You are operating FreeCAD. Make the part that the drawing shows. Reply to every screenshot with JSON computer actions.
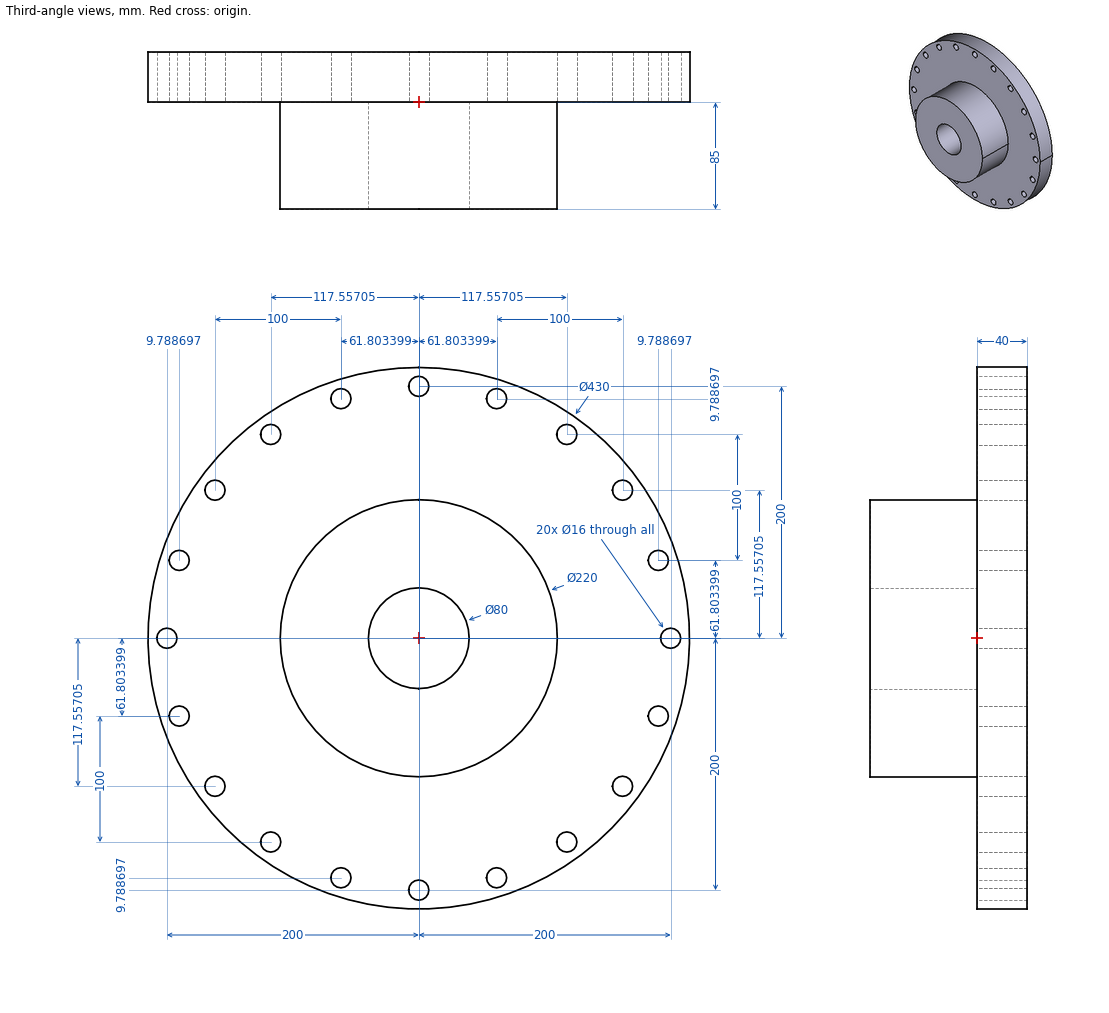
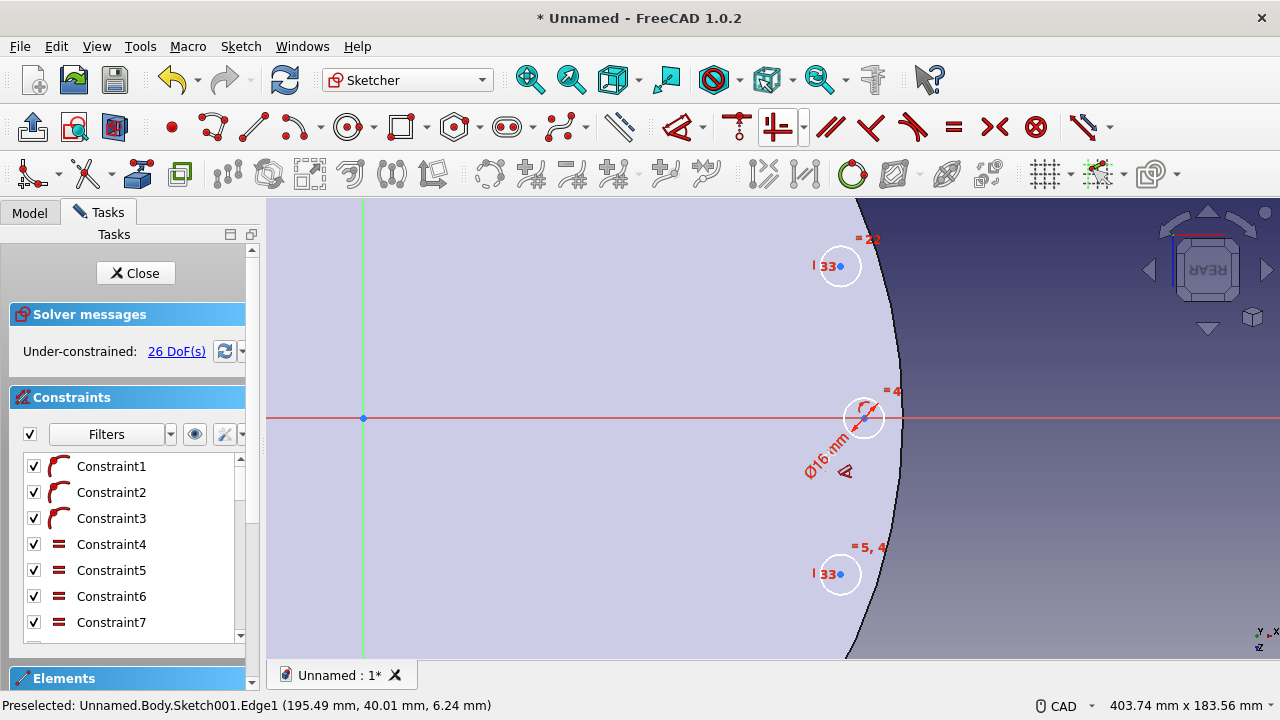
{"action": "left_click", "coordinate": [864, 418]}
{"action": "left_click", "coordinate": [614, 452]}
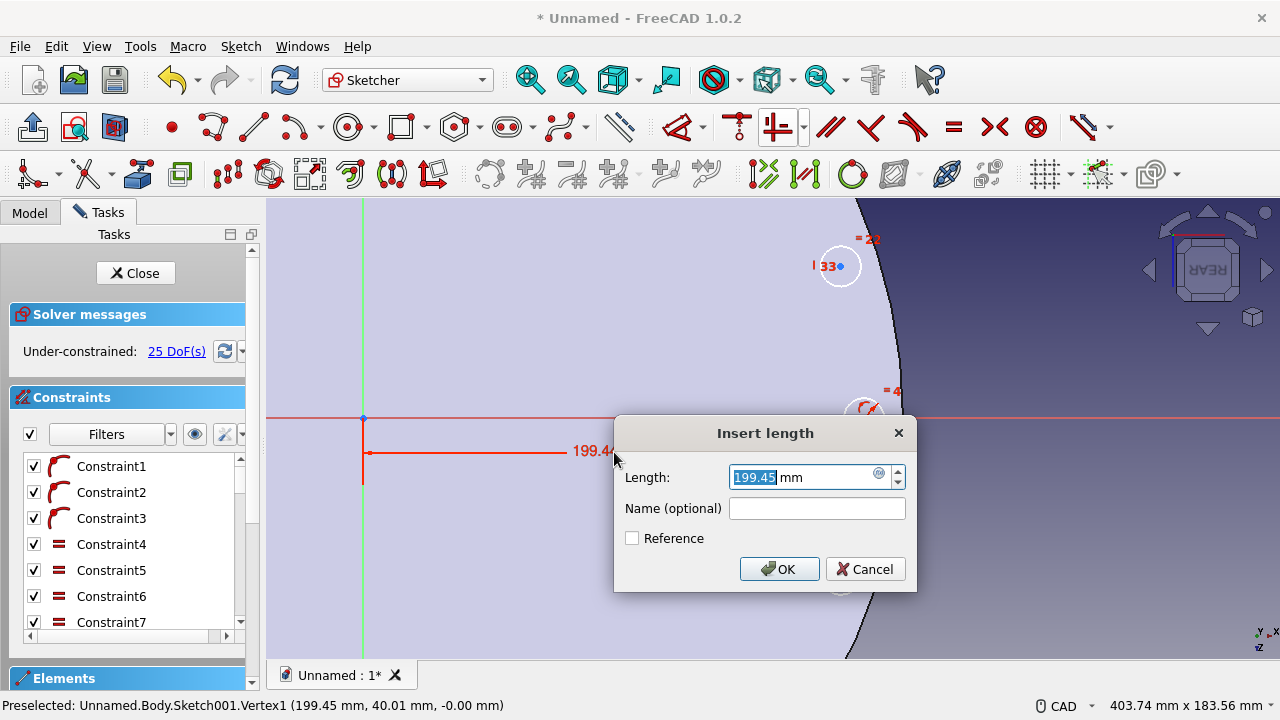
{"action": "type", "text": "200"}
{"action": "key", "text": "Return"}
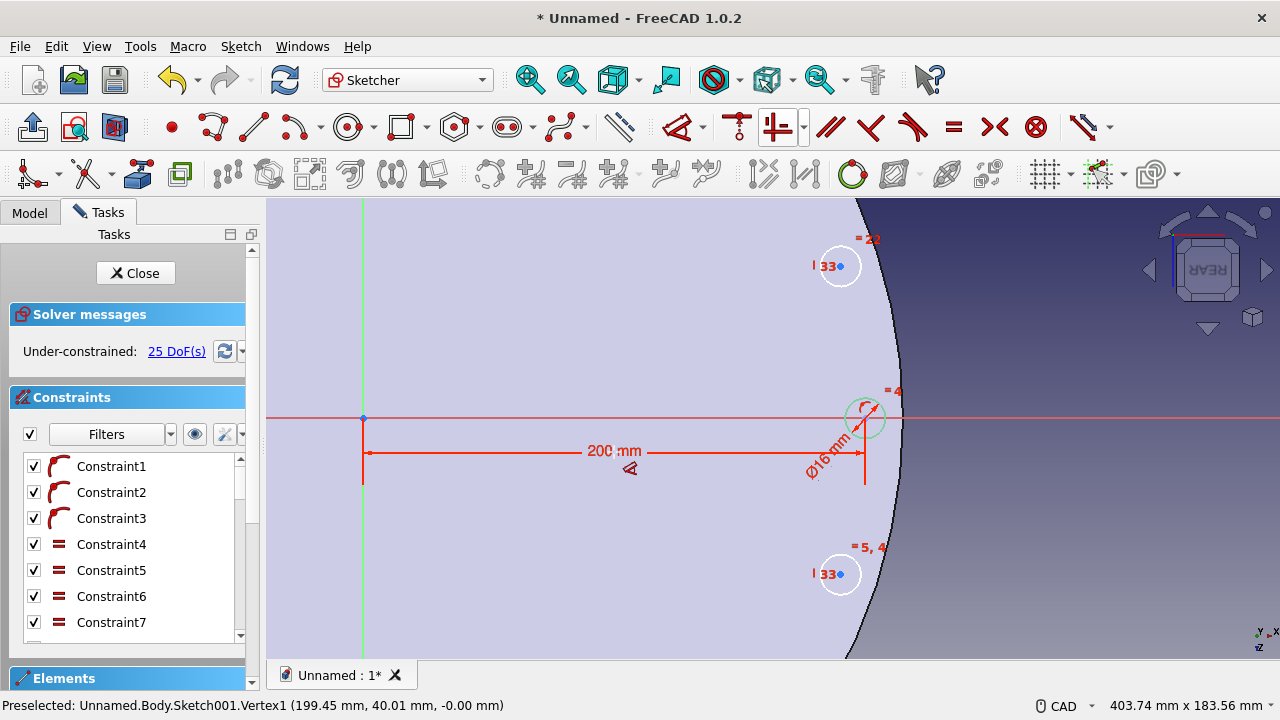
{"action": "scroll", "coordinate": [852, 433], "scroll_direction": "down", "scroll_amount": 6}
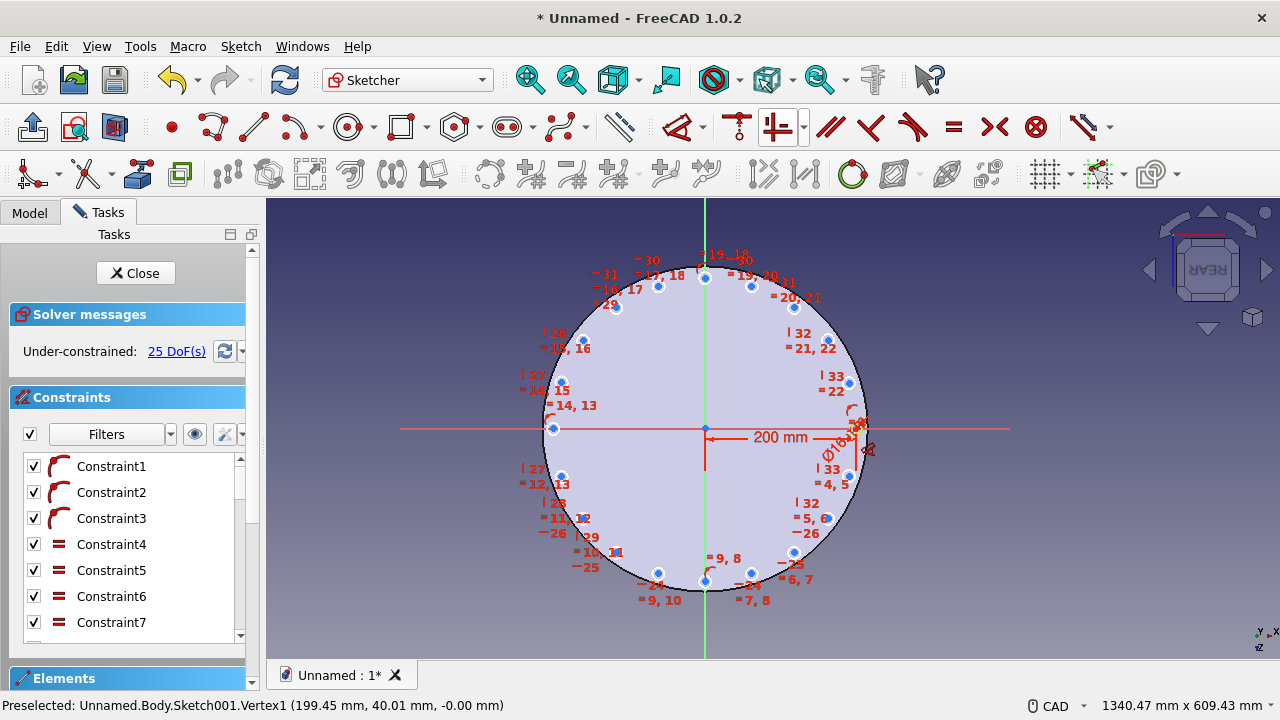
{"action": "left_click", "coordinate": [705, 582]}
{"action": "left_click", "coordinate": [739, 505]}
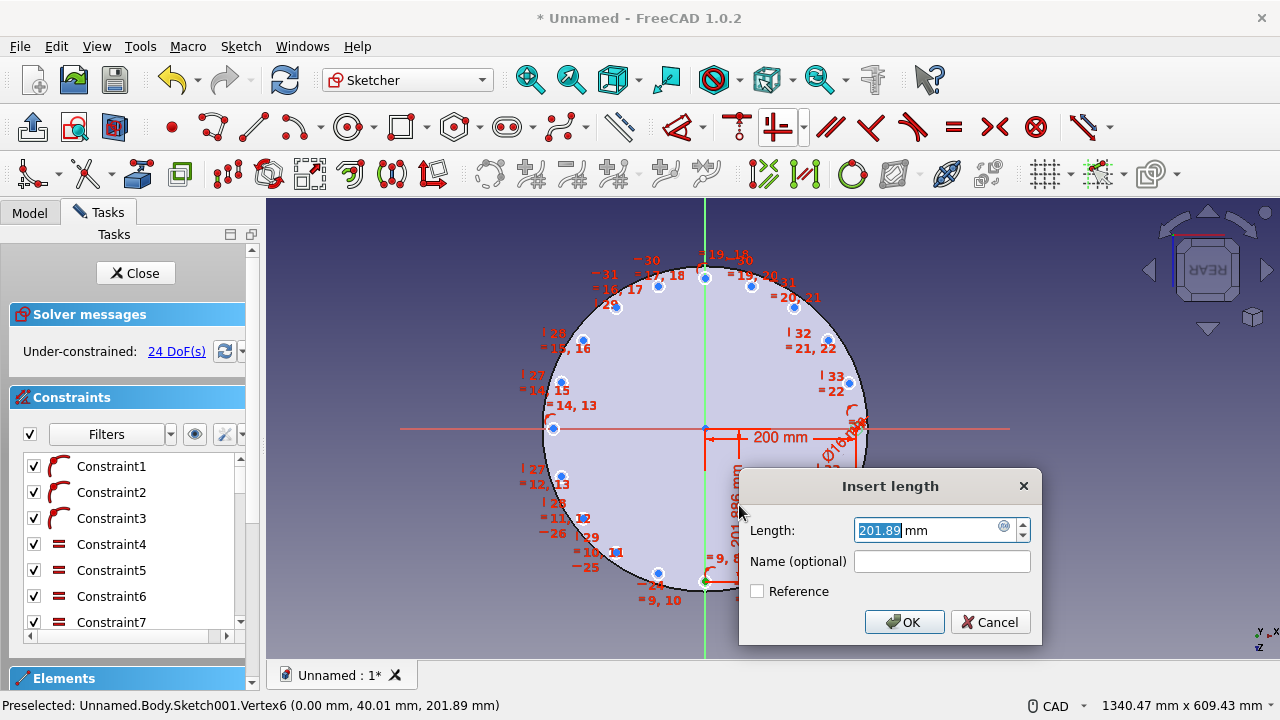
{"action": "type", "text": "200"}
{"action": "key", "text": "Return"}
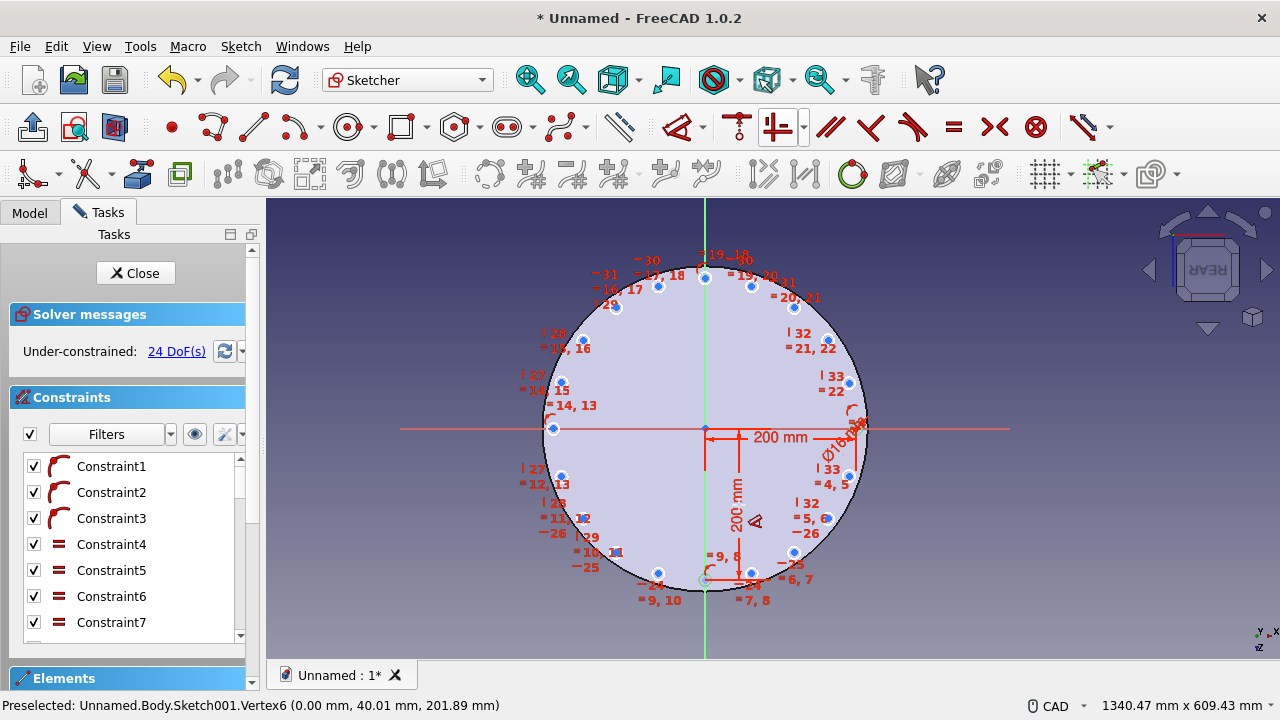
{"action": "left_click", "coordinate": [553, 429]}
{"action": "left_click", "coordinate": [629, 463]}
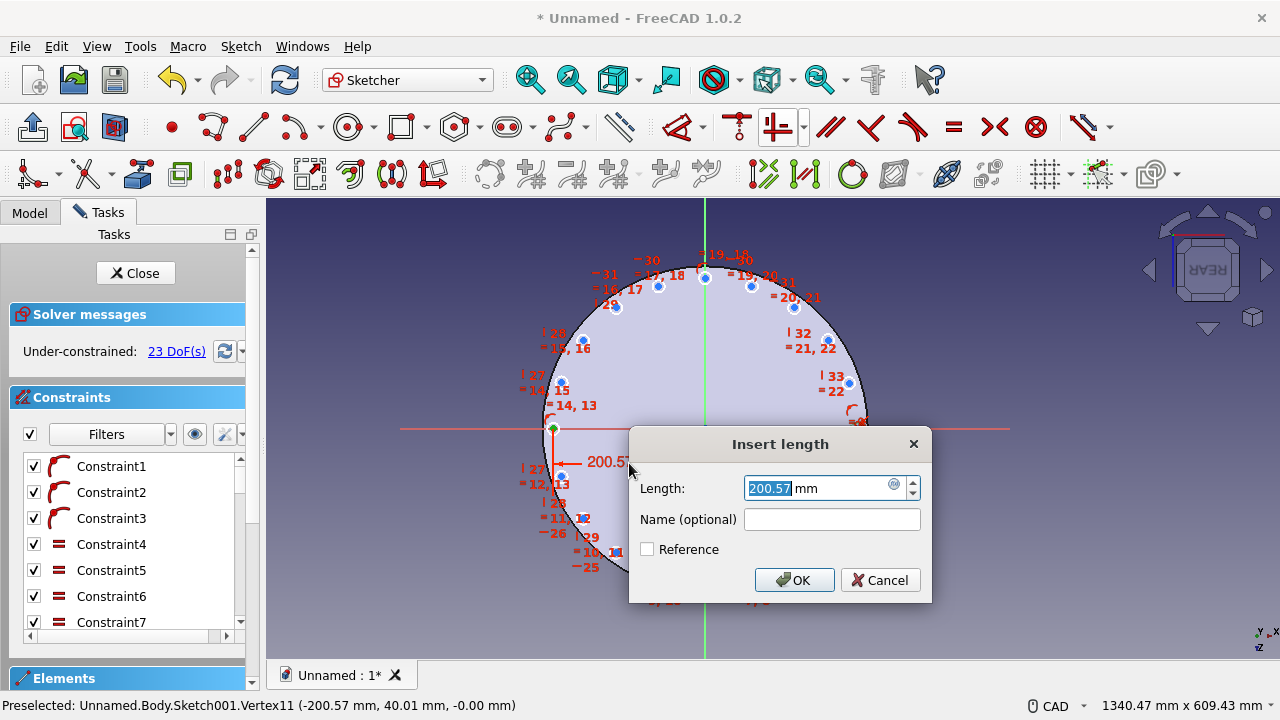
{"action": "type", "text": "200"}
{"action": "key", "text": "Return"}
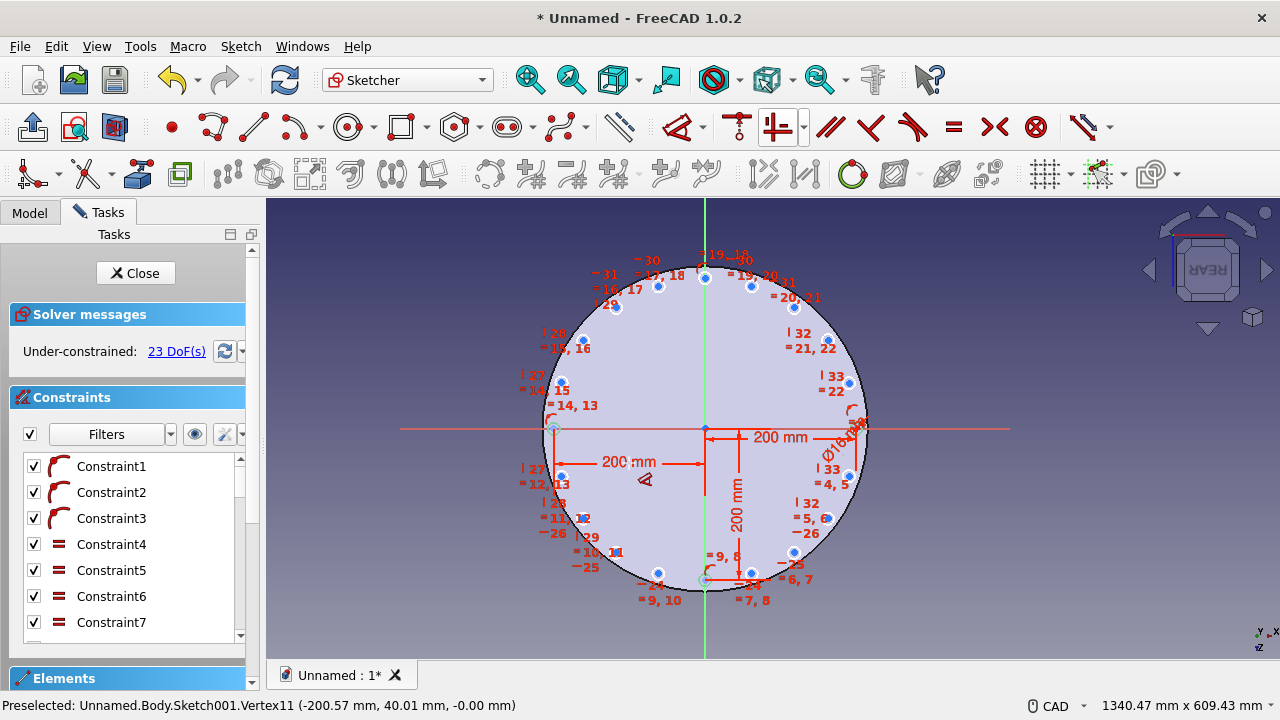
{"action": "left_click", "coordinate": [705, 278]}
{"action": "left_click", "coordinate": [739, 354]}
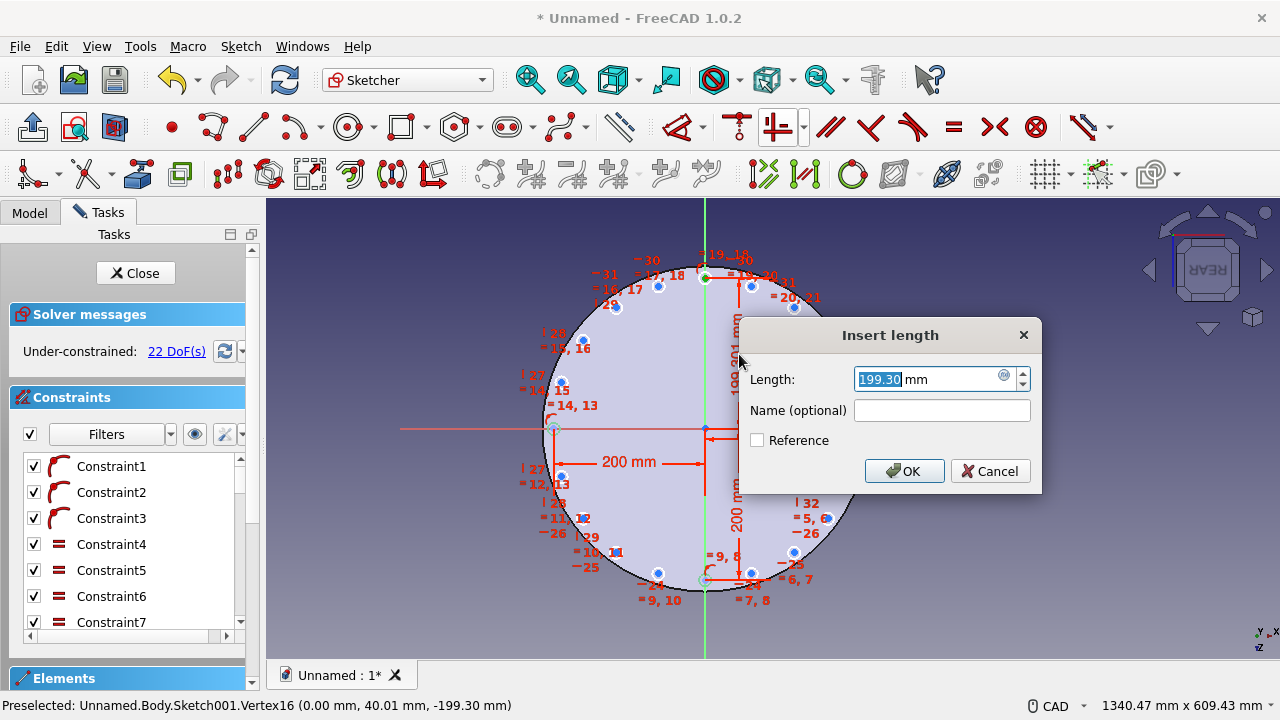
{"action": "type", "text": "200"}
{"action": "key", "text": "Return"}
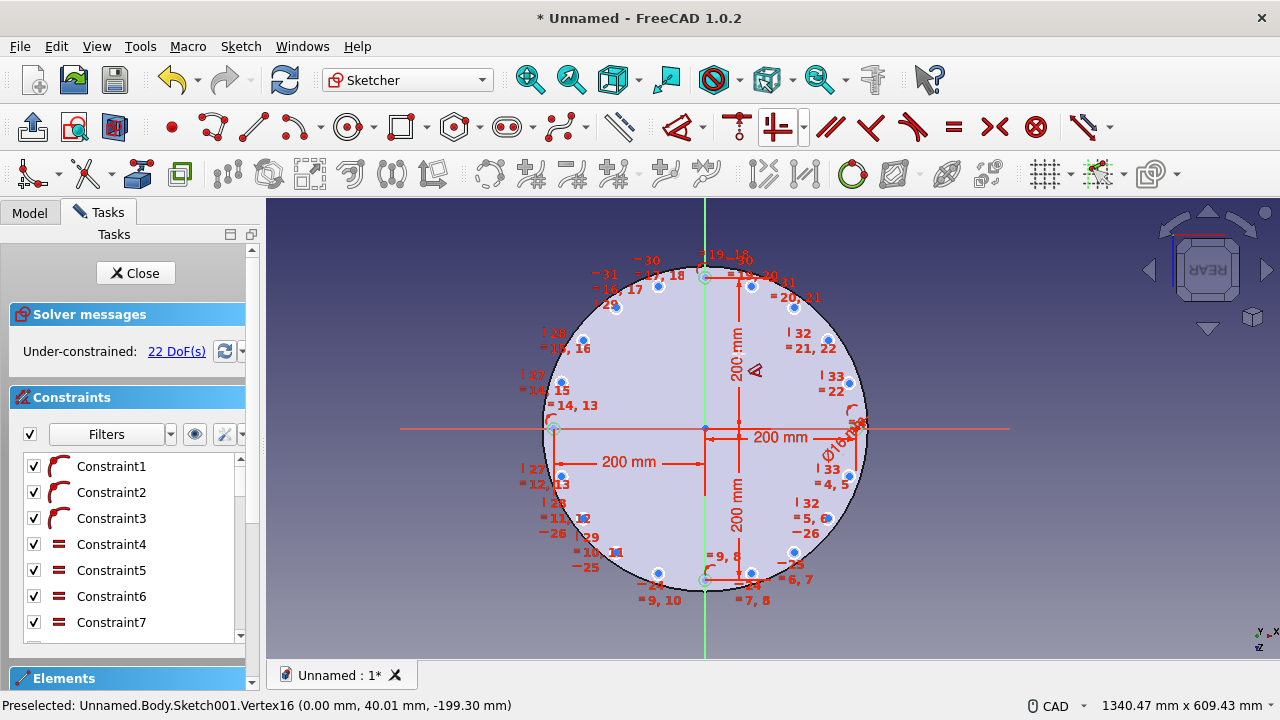
{"action": "left_click", "coordinate": [849, 476]}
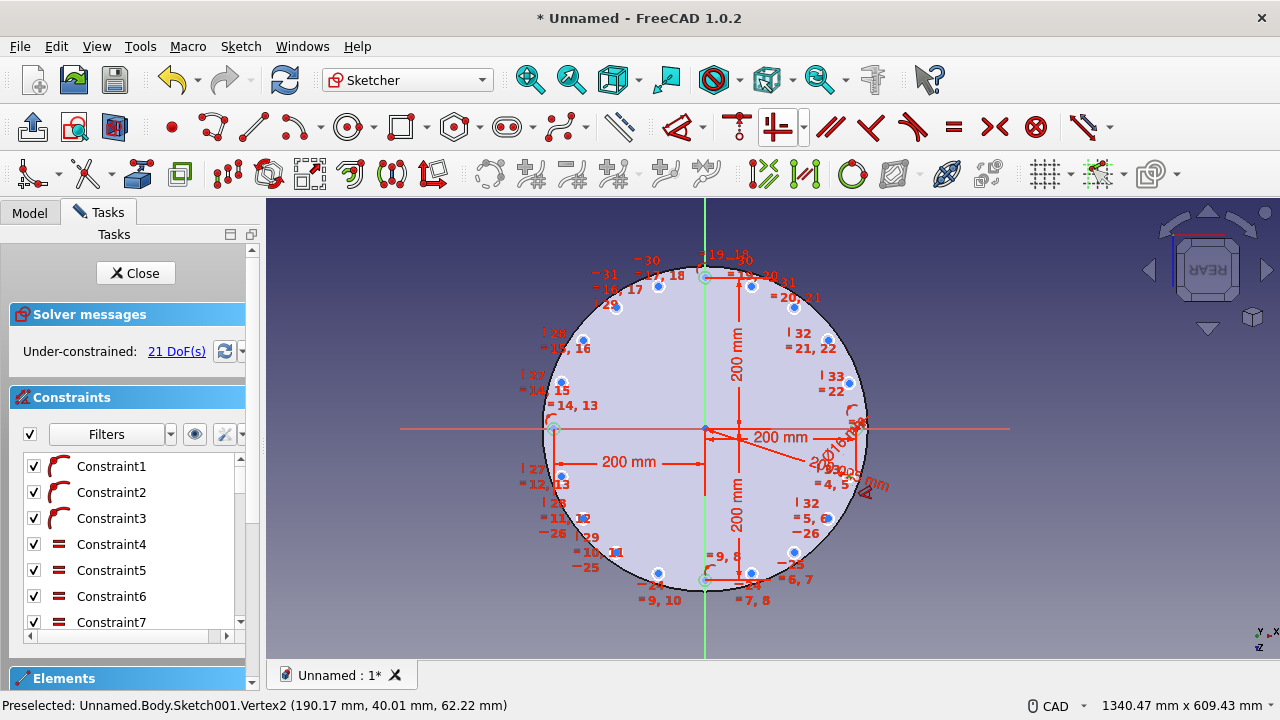
{"action": "left_click", "coordinate": [794, 553]}
{"action": "left_click", "coordinate": [883, 514]}